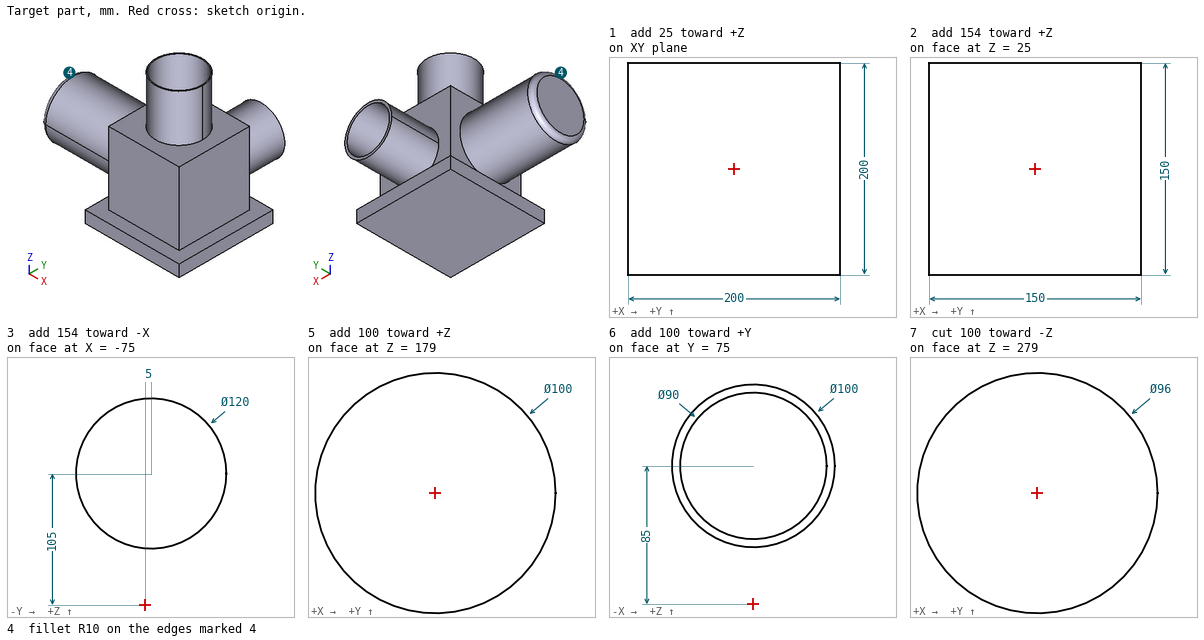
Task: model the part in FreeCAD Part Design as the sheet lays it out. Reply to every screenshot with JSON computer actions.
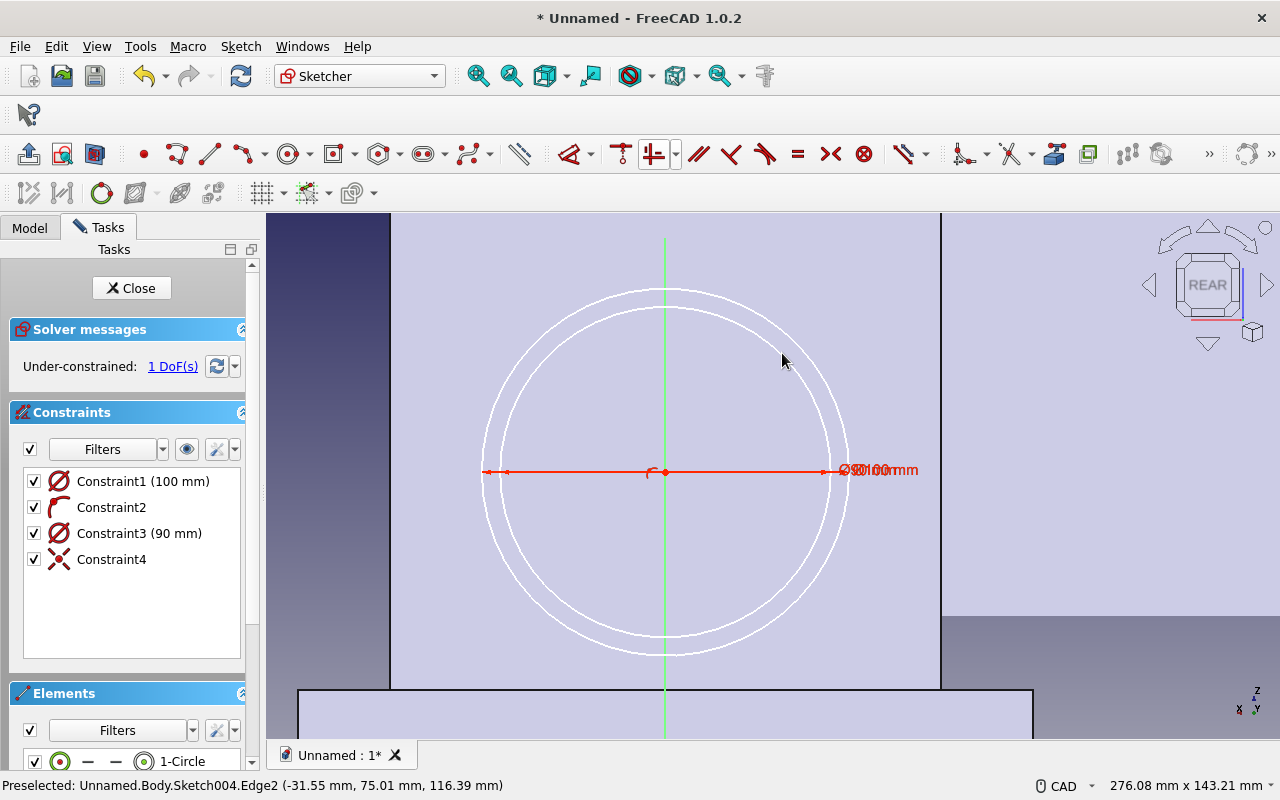
{"action": "left_click", "coordinate": [568, 154]}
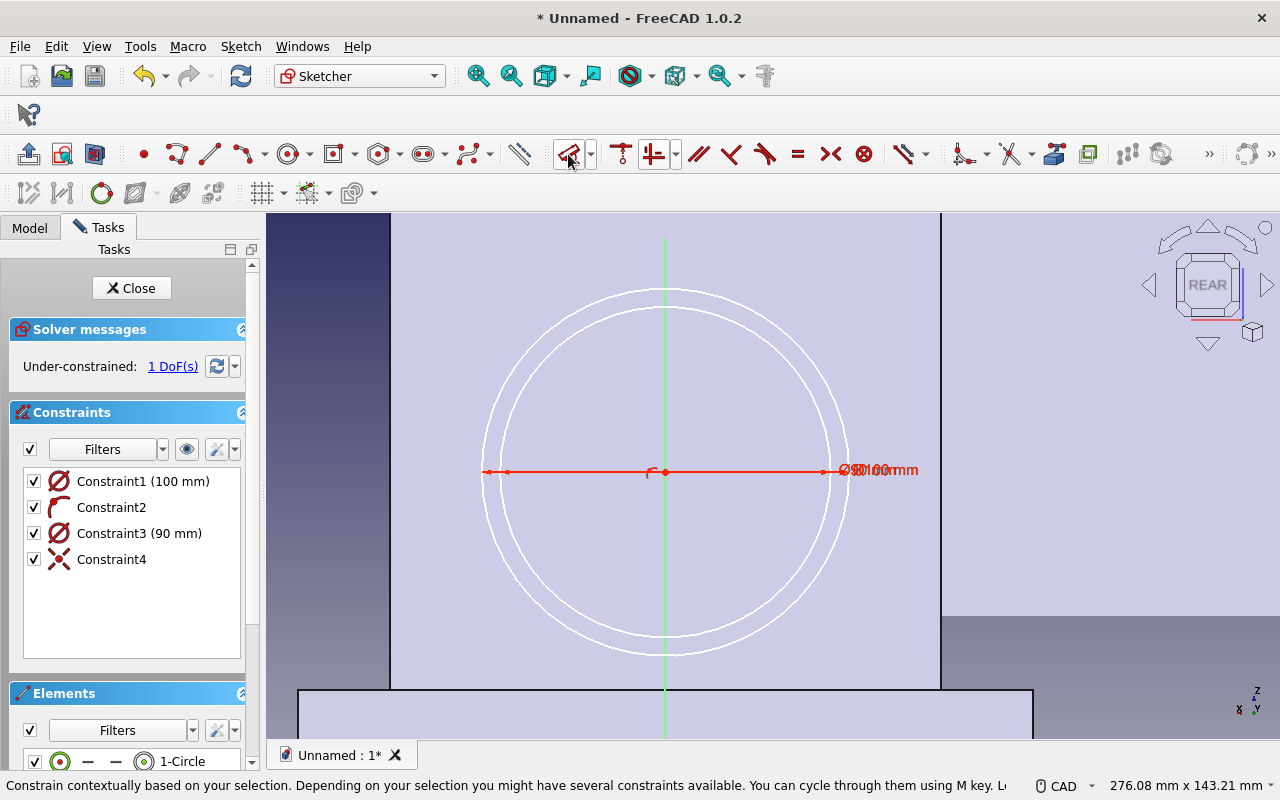
{"action": "left_click", "coordinate": [665, 472]}
{"action": "left_click", "coordinate": [699, 592]}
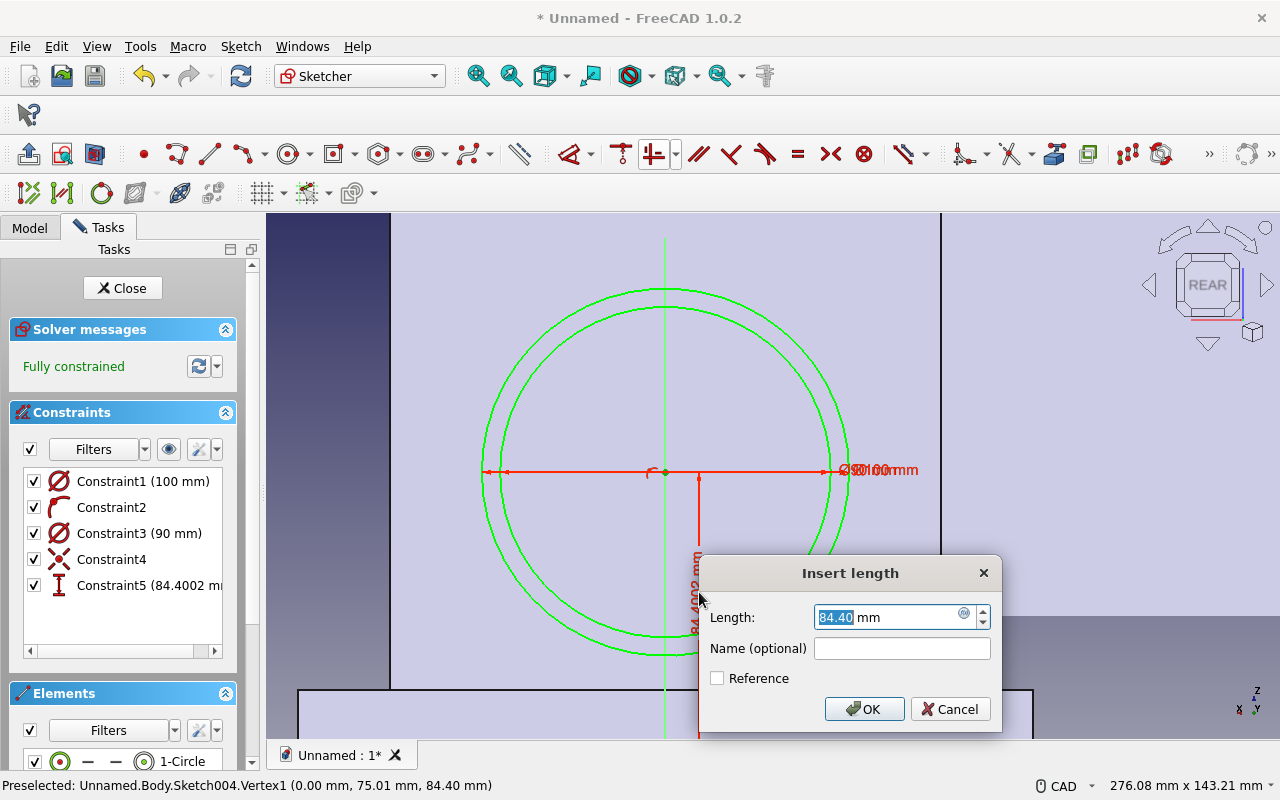
{"action": "type", "text": "85"}
{"action": "key", "text": "Return"}
{"action": "key", "text": "Escape"}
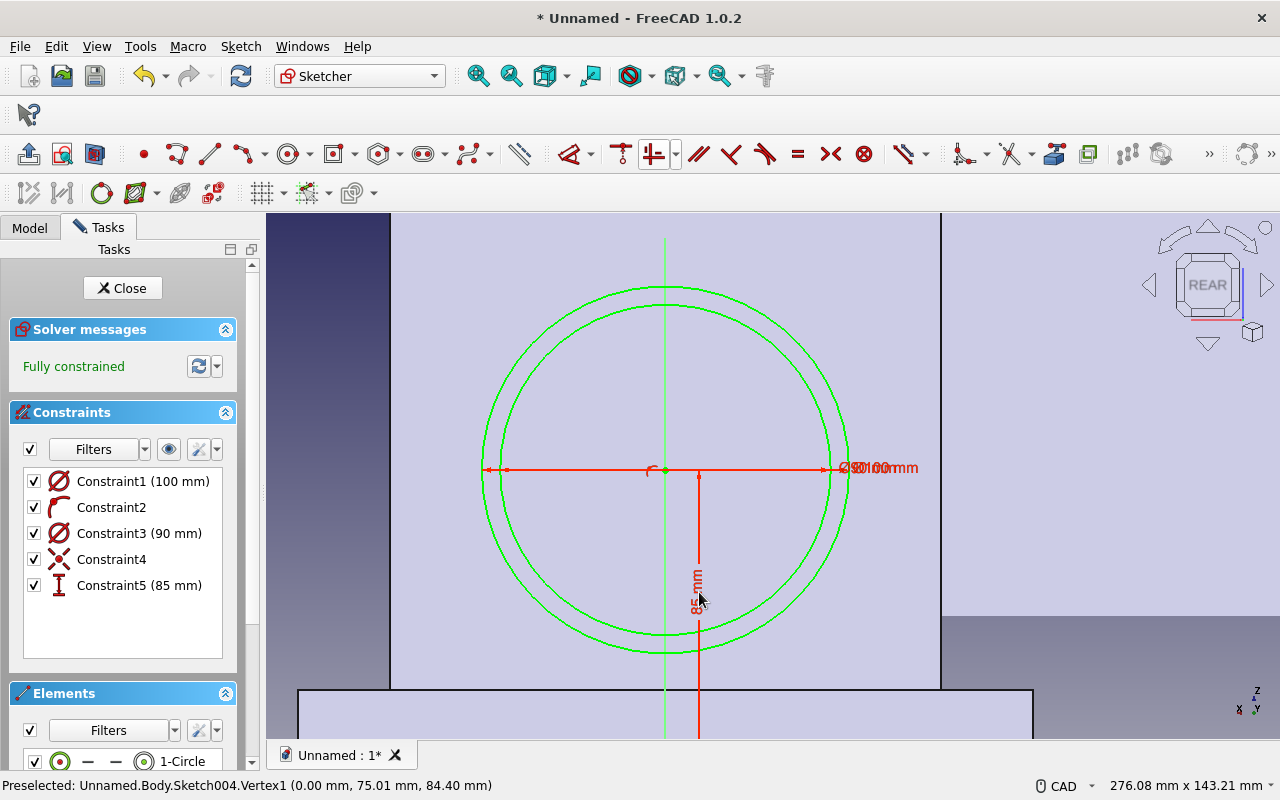
{"action": "left_click", "coordinate": [123, 288]}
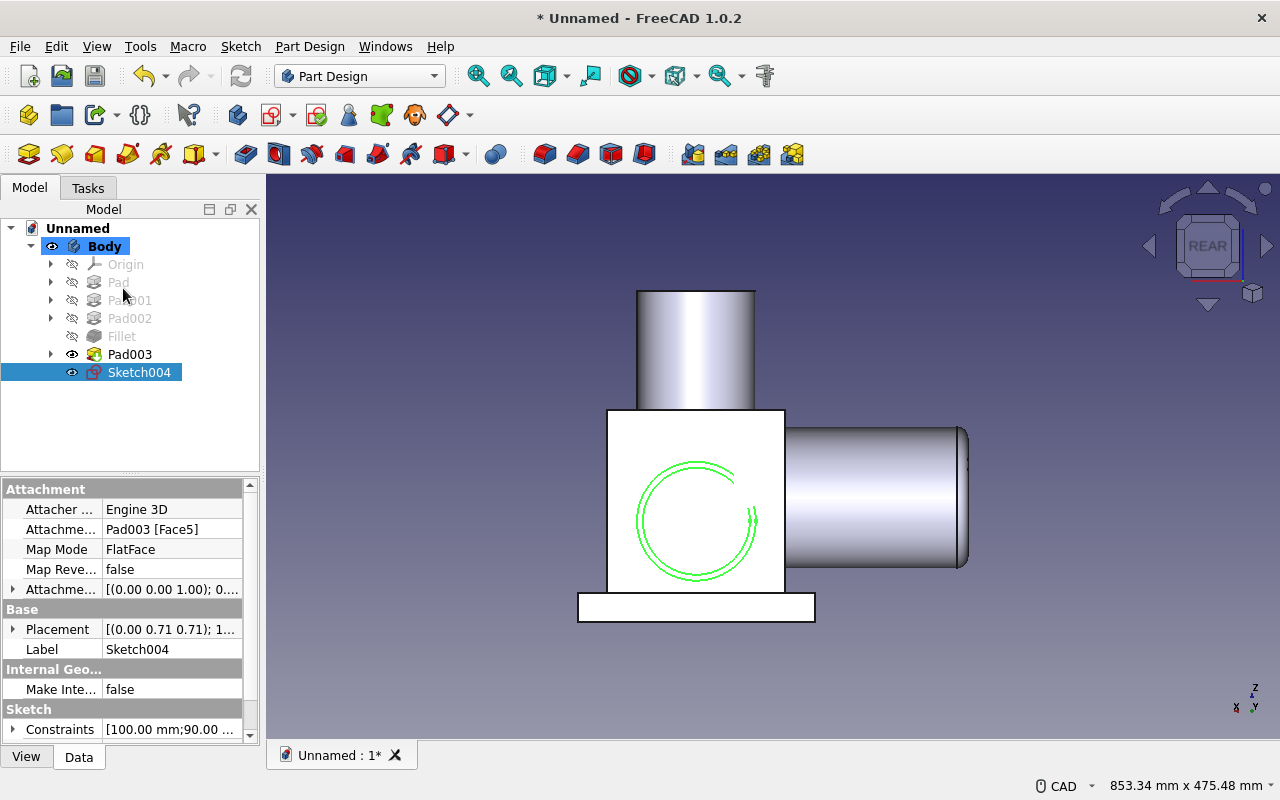
{"action": "left_click", "coordinate": [29, 154]}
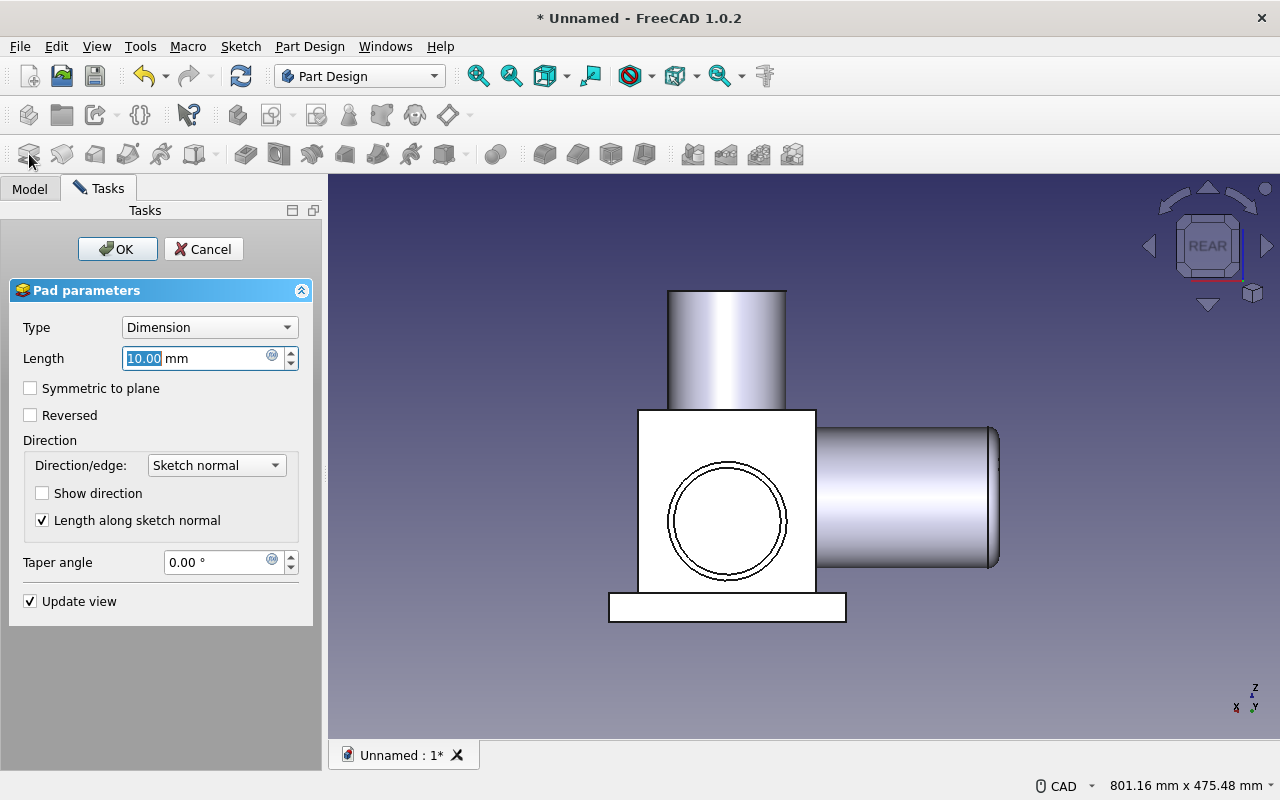
{"action": "type", "text": "100"}
{"action": "key", "text": "Tab"}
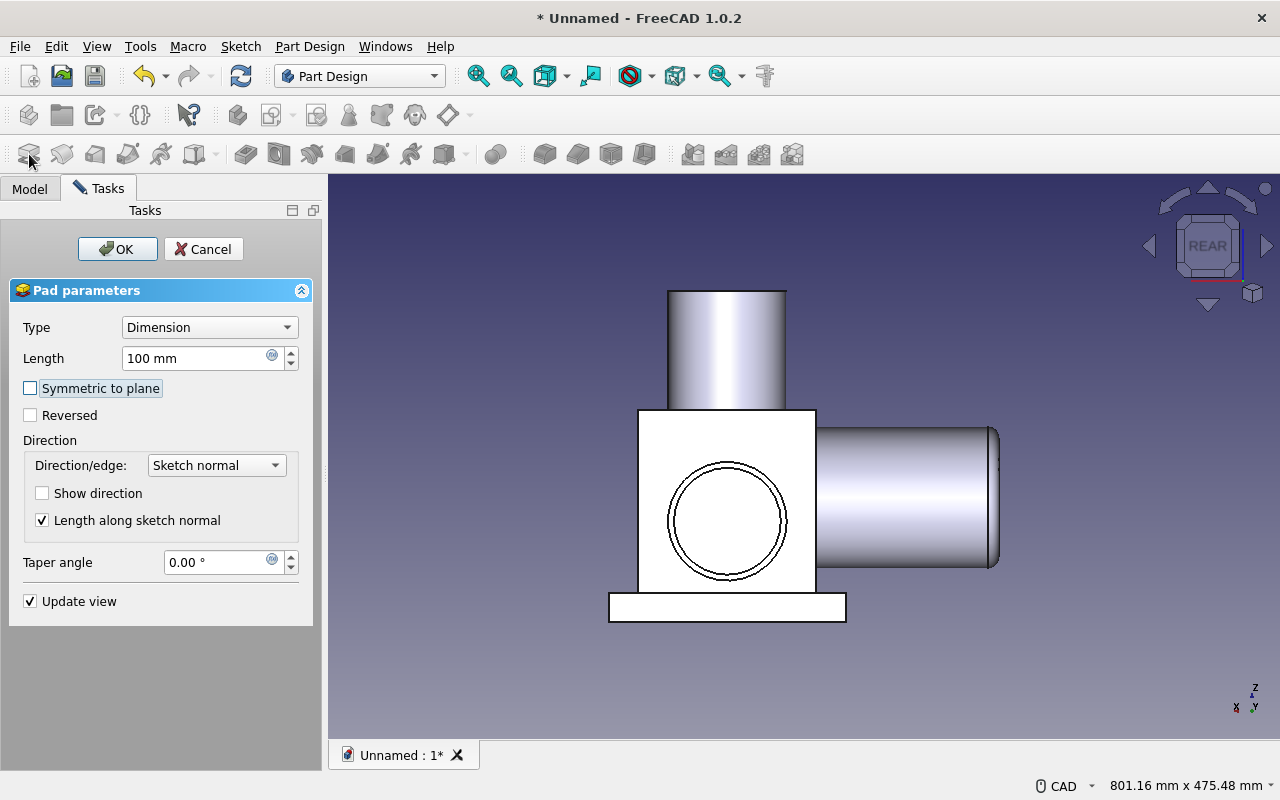
{"action": "left_click", "coordinate": [118, 249]}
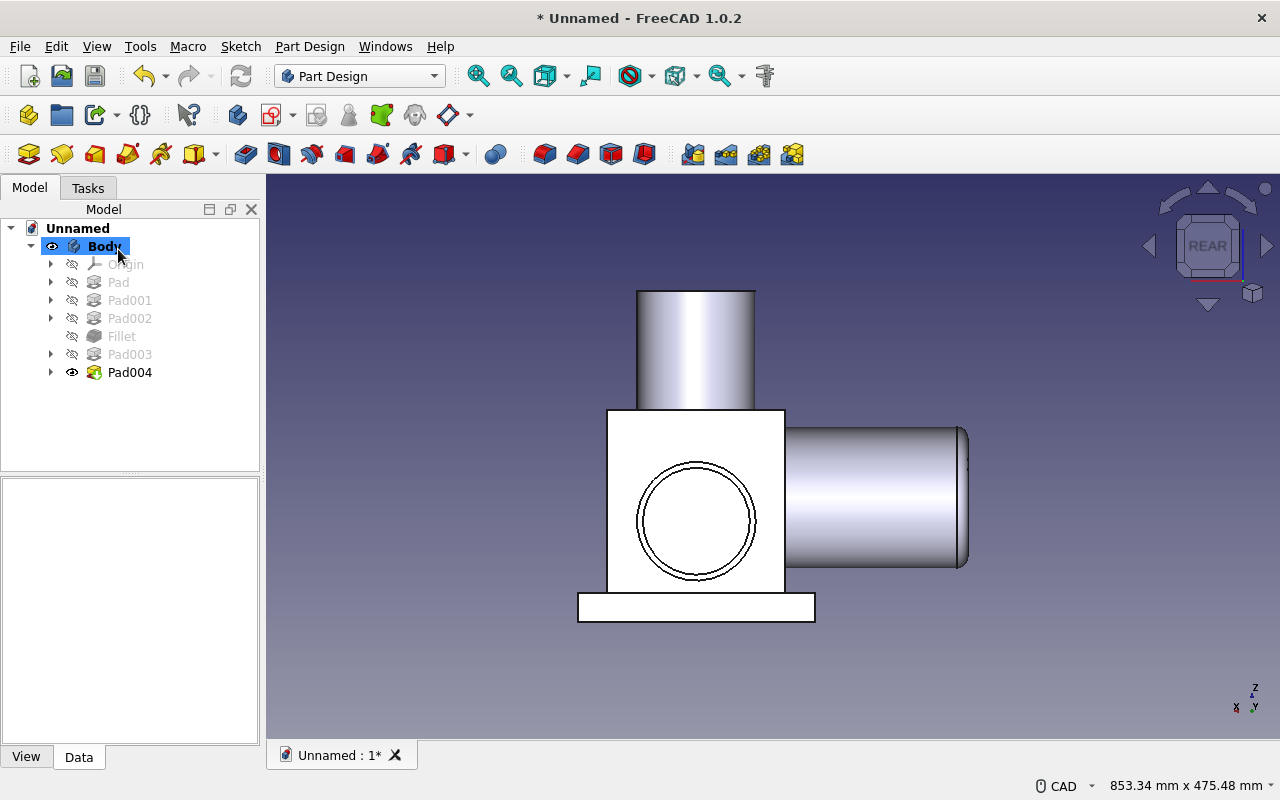
{"action": "key", "text": "0"}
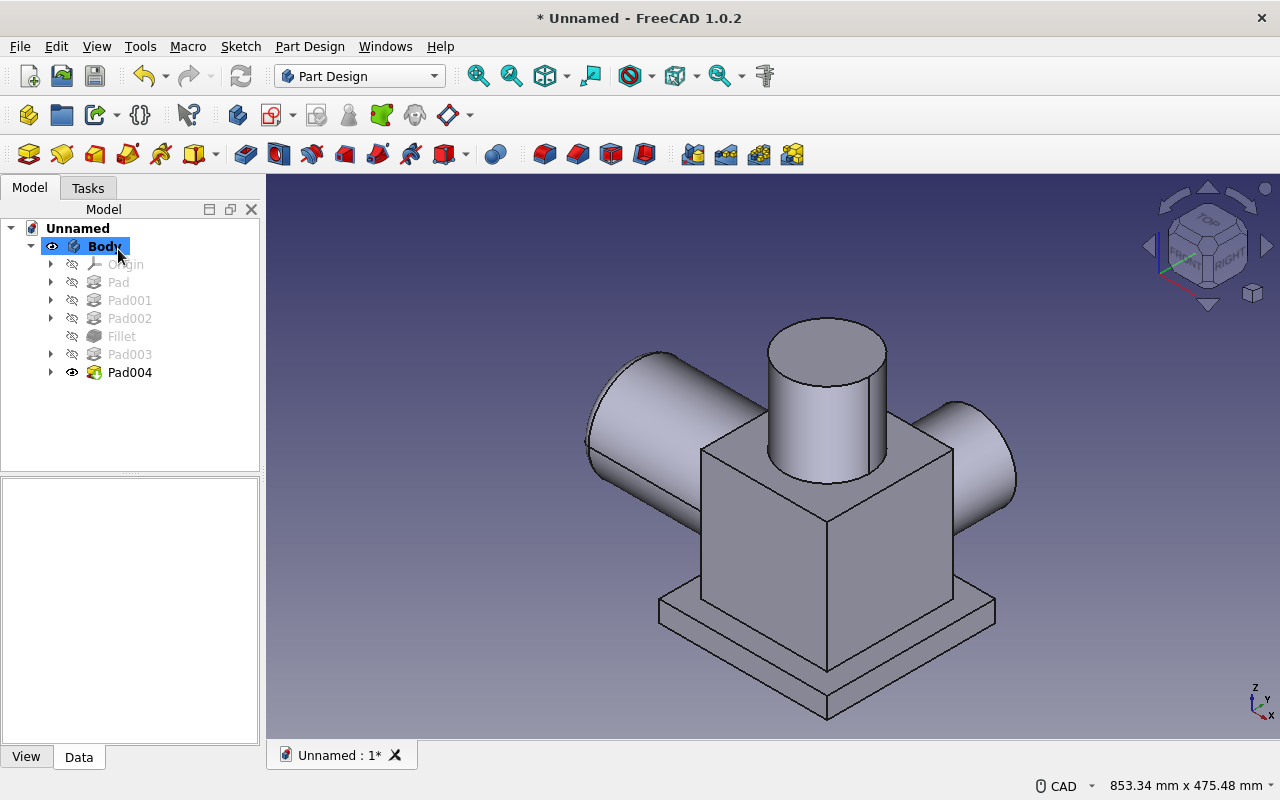
{"action": "left_click", "coordinate": [479, 76]}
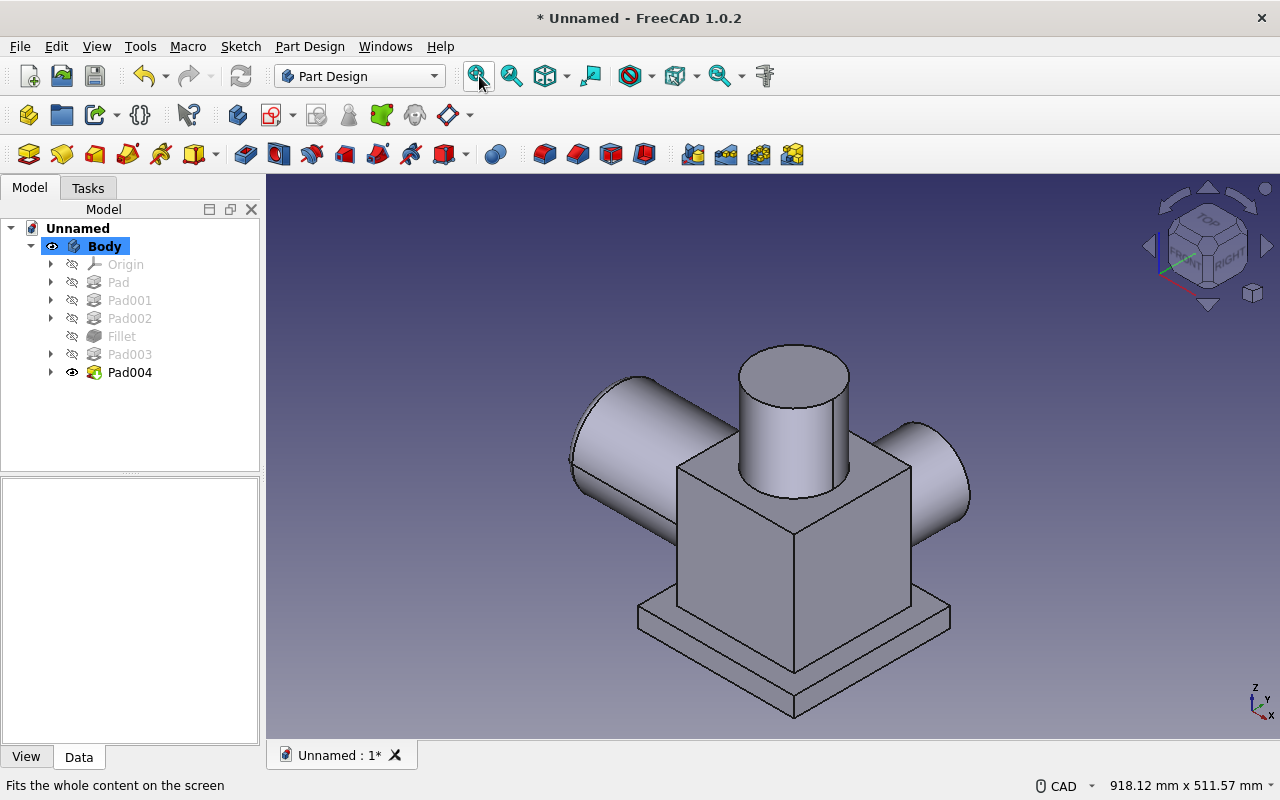
{"action": "left_click", "coordinate": [794, 376]}